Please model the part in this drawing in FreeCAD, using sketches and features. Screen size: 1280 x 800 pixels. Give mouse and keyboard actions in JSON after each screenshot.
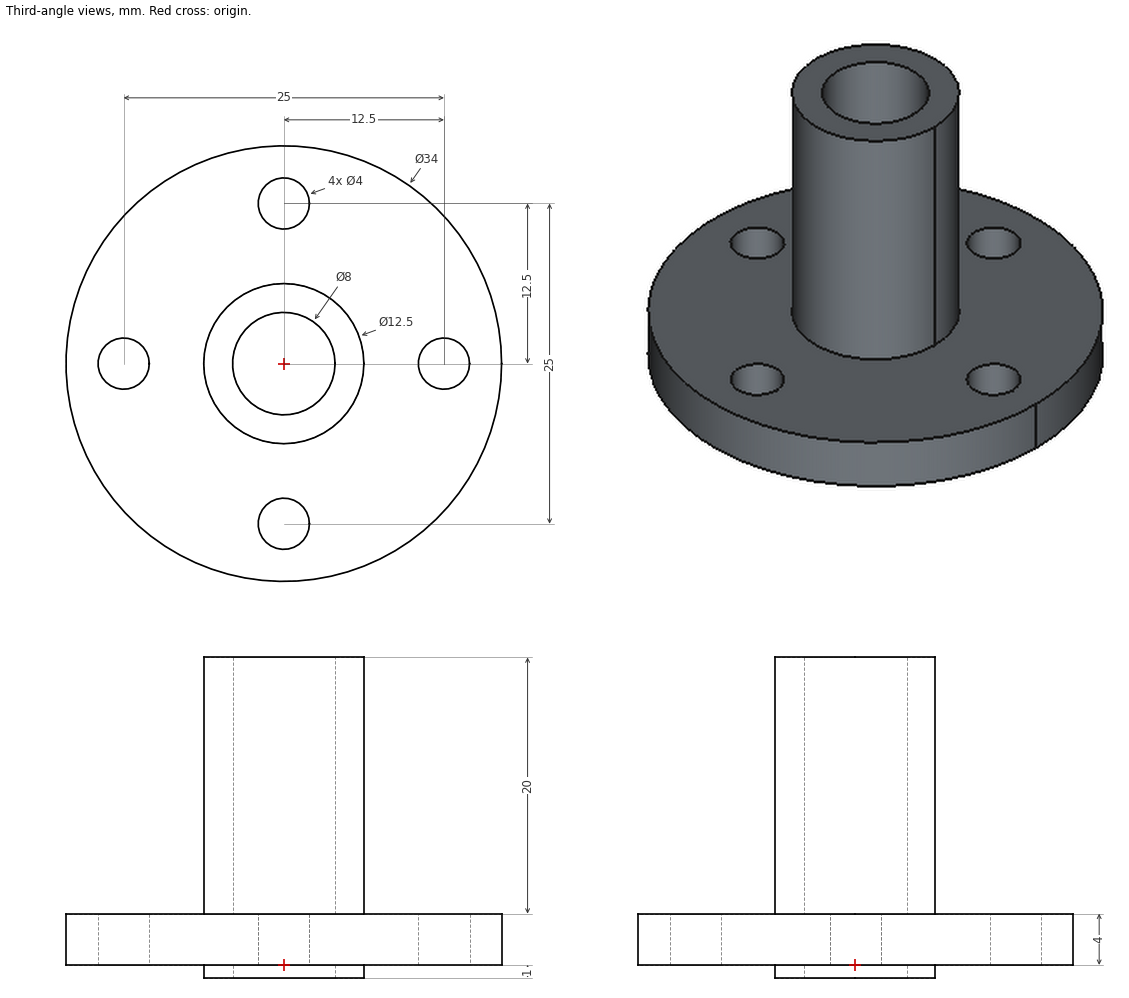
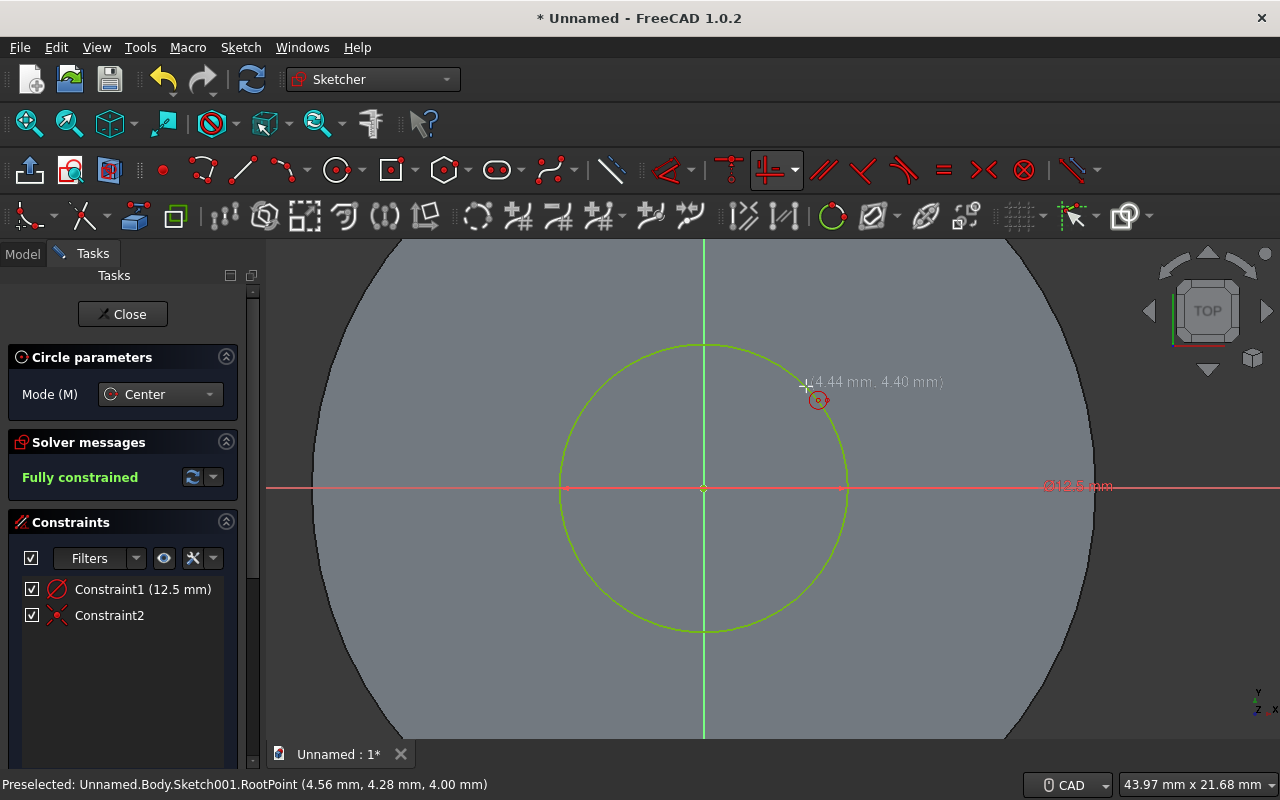
{"action": "left_click", "coordinate": [704, 488]}
{"action": "mouse_move", "coordinate": [769, 423]}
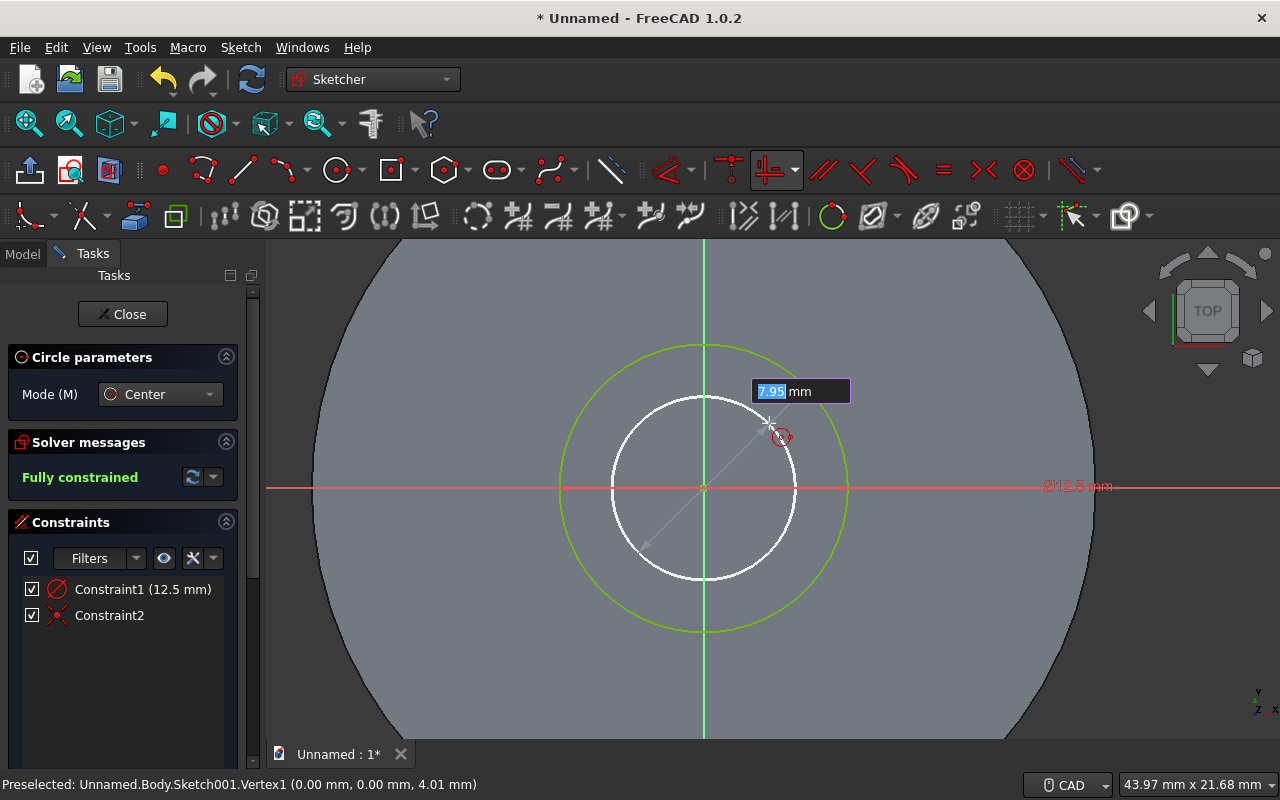
{"action": "type", "text": "8"}
{"action": "key", "text": "Return"}
{"action": "key", "text": "Escape"}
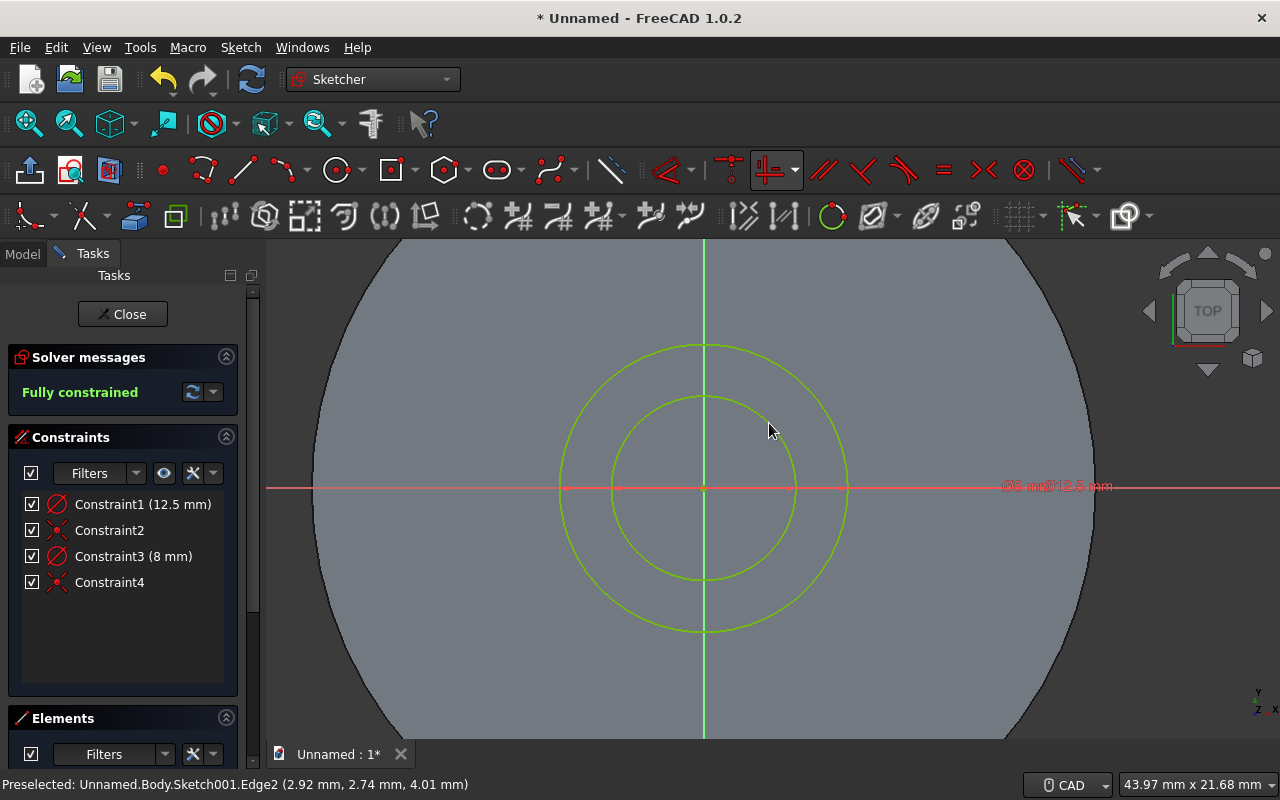
{"action": "left_click", "coordinate": [123, 314]}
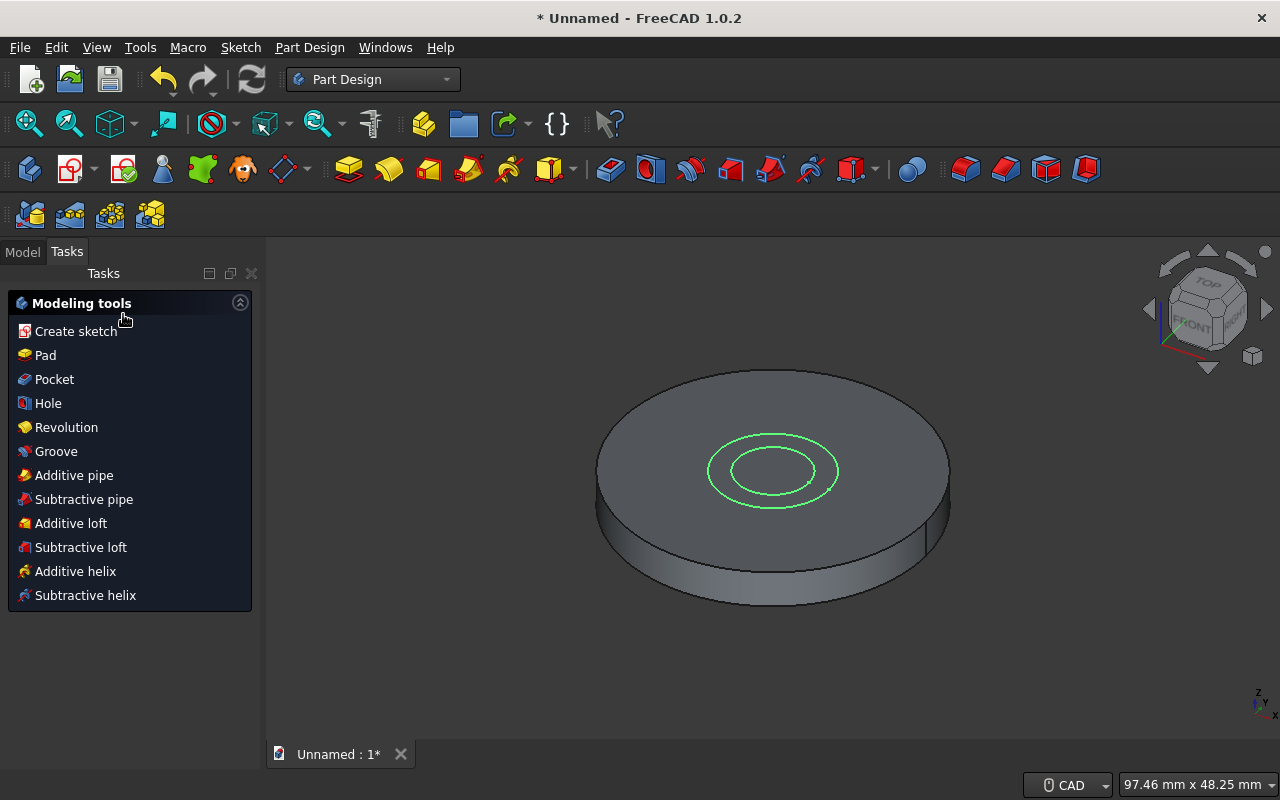
{"action": "left_click", "coordinate": [350, 170]}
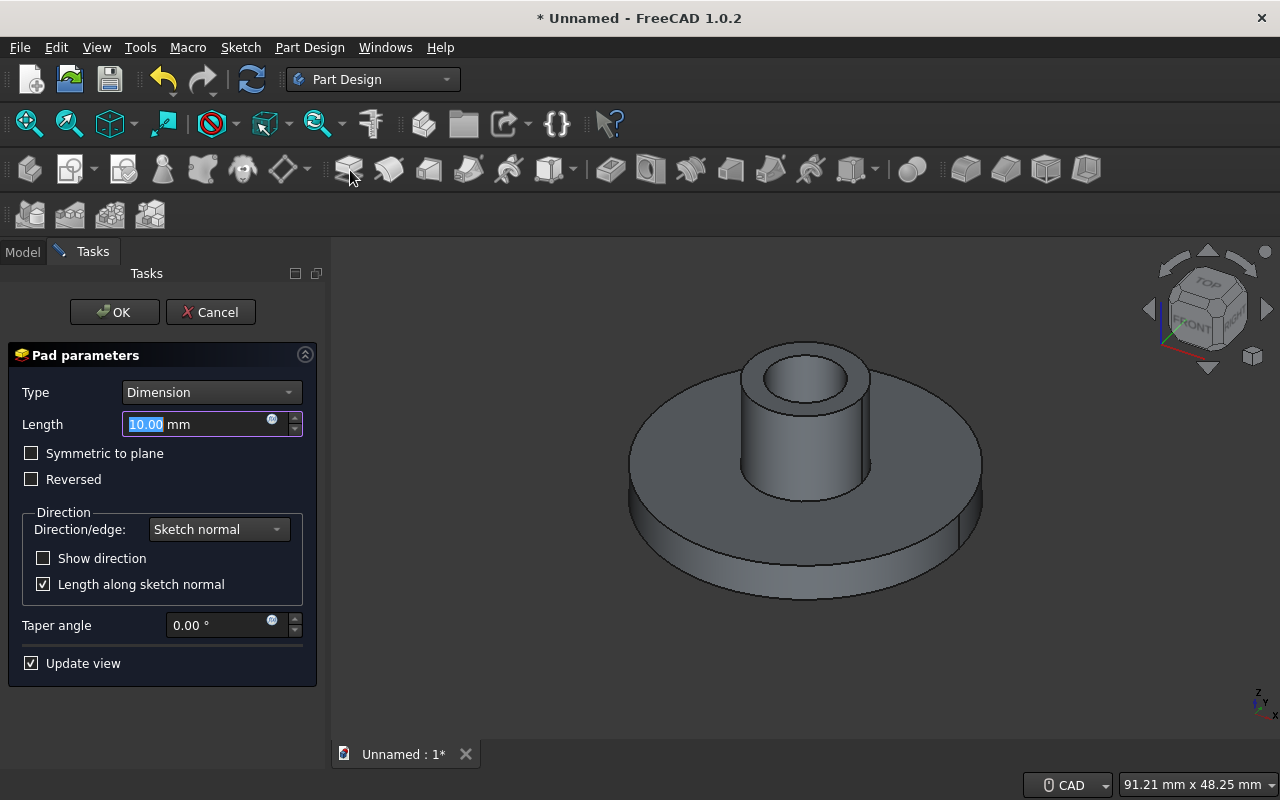
{"action": "type", "text": "20"}
{"action": "key", "text": "Tab"}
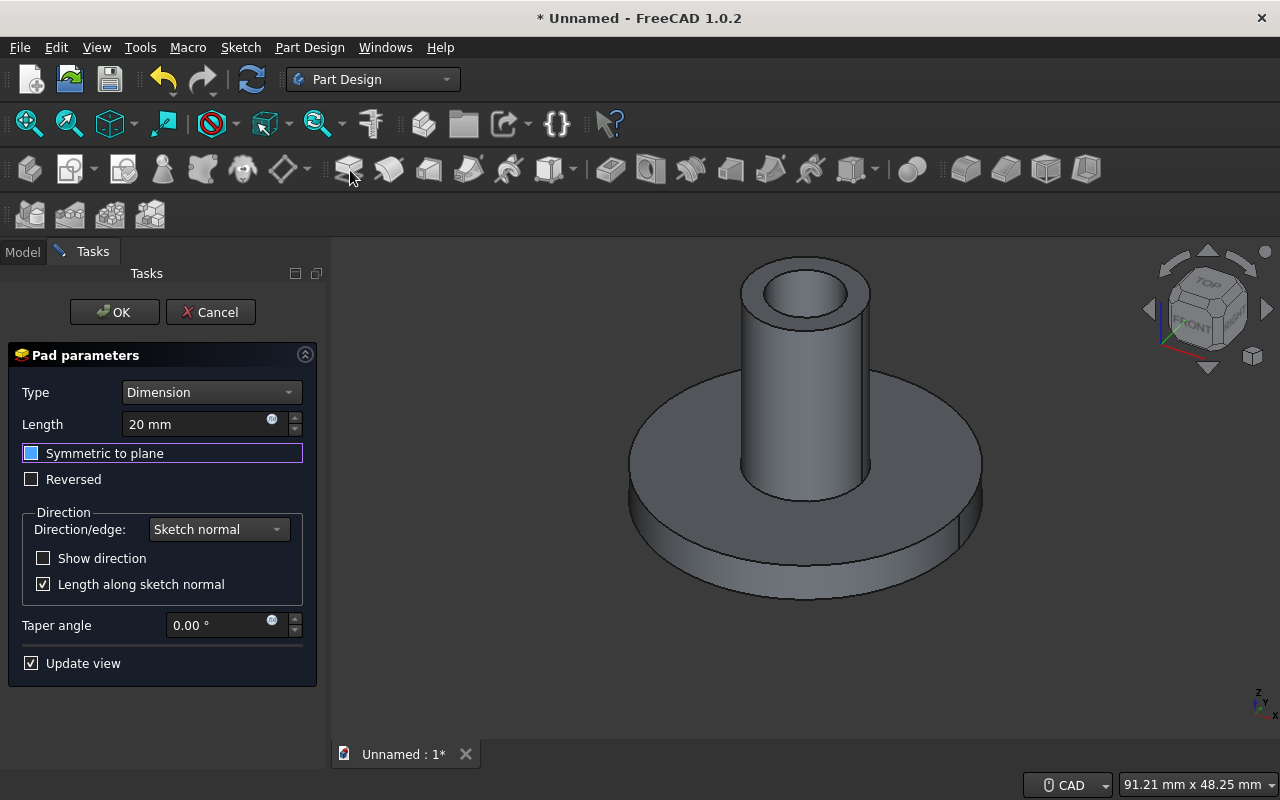
{"action": "left_click", "coordinate": [115, 312]}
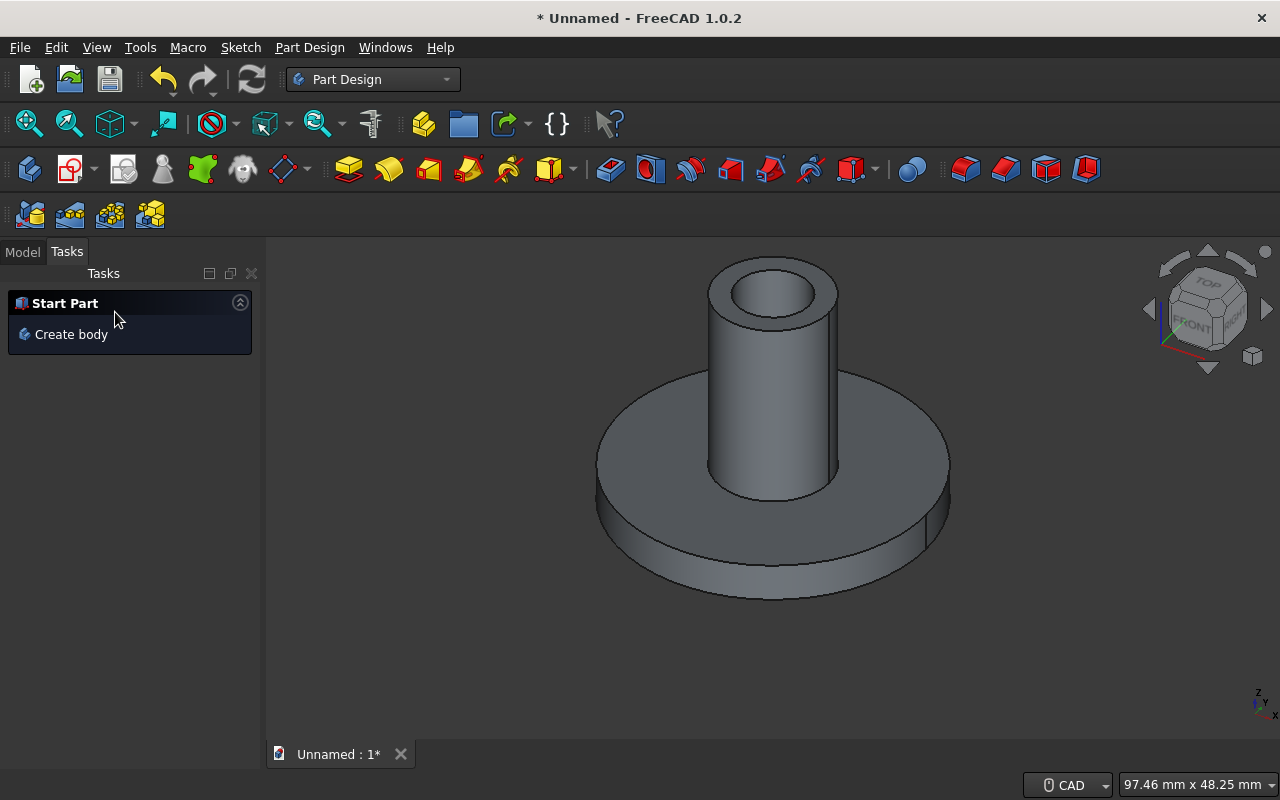
{"action": "left_click", "coordinate": [30, 124]}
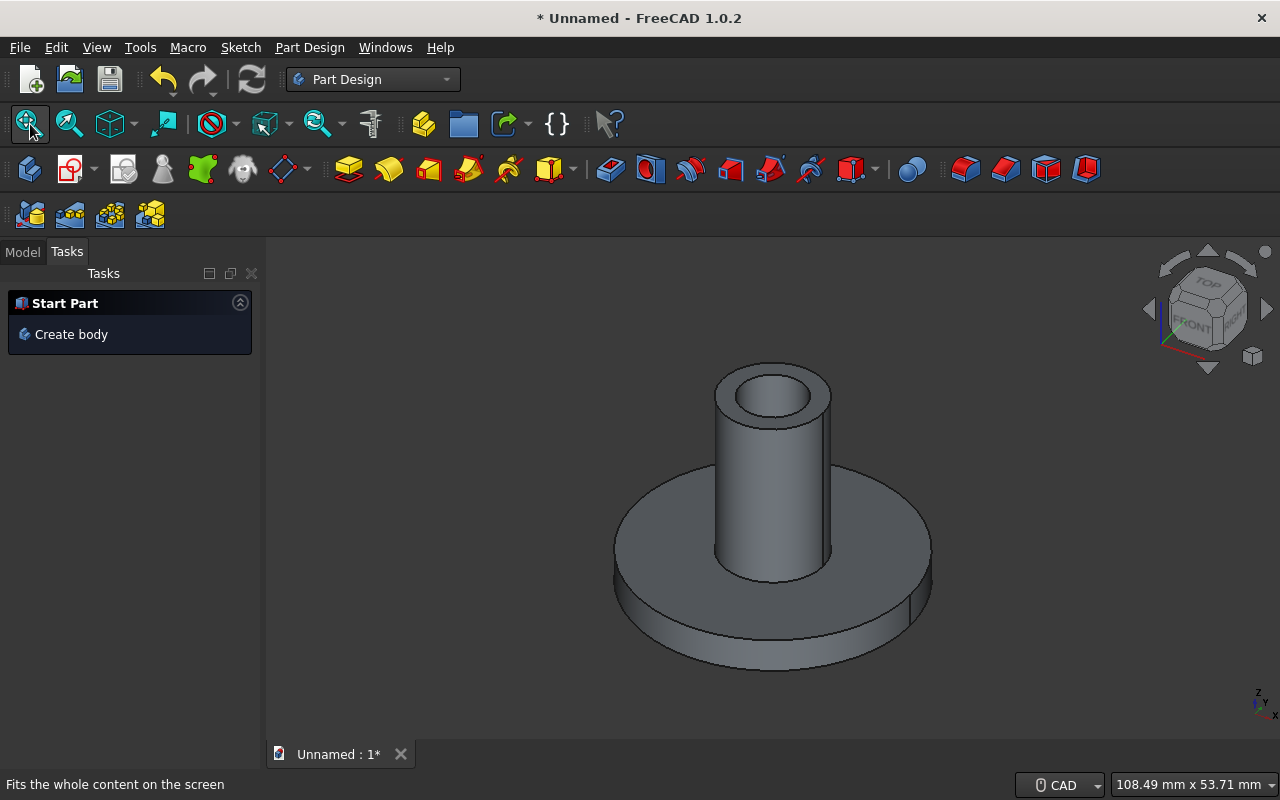
{"action": "left_click", "coordinate": [858, 516]}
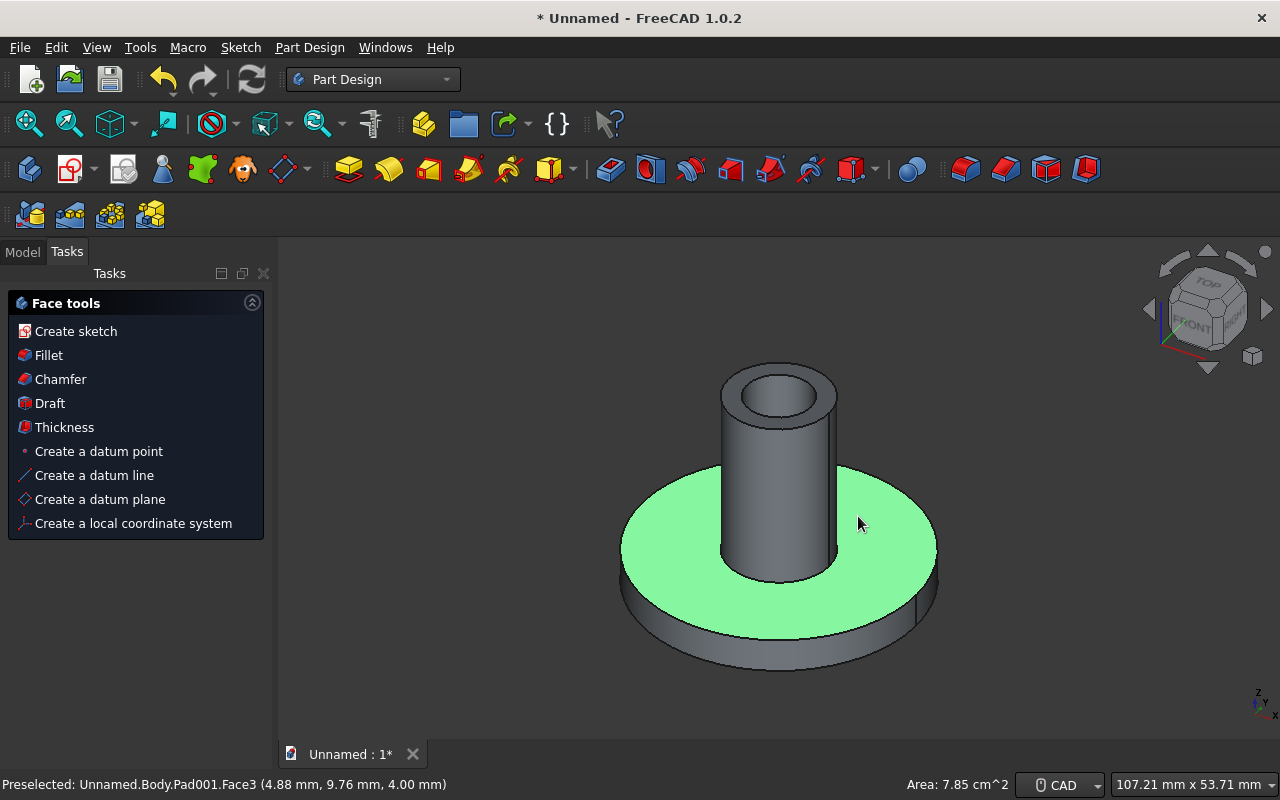
{"action": "left_click", "coordinate": [70, 170]}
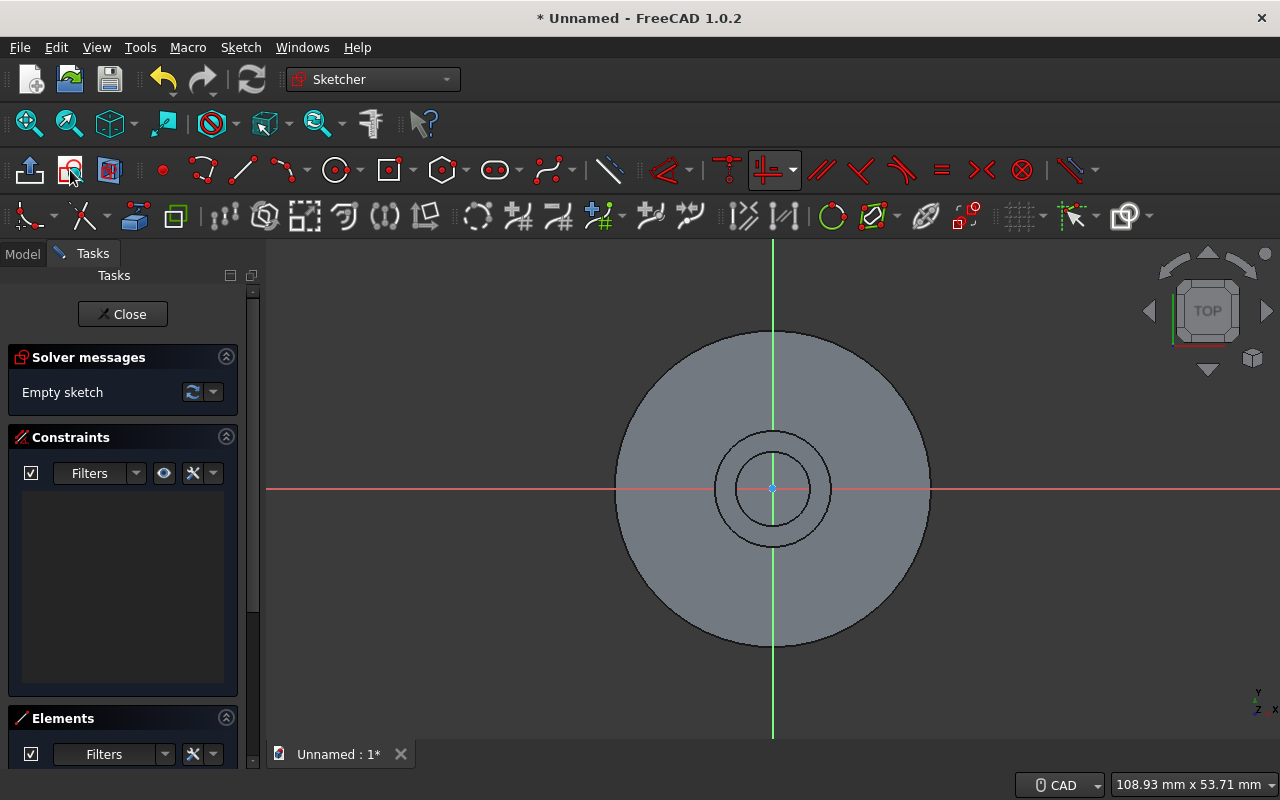
{"action": "left_click", "coordinate": [110, 170]}